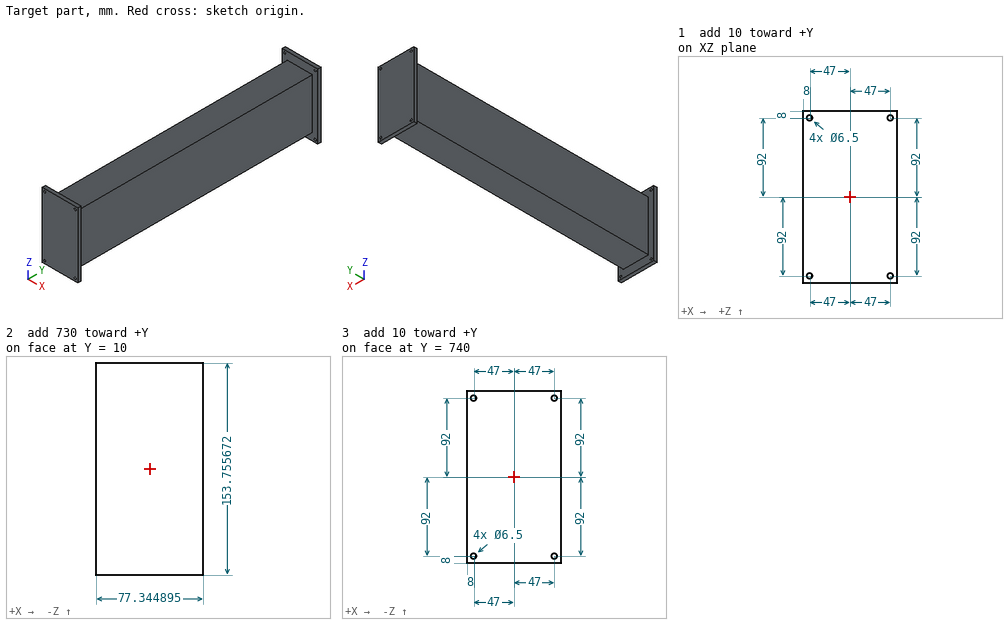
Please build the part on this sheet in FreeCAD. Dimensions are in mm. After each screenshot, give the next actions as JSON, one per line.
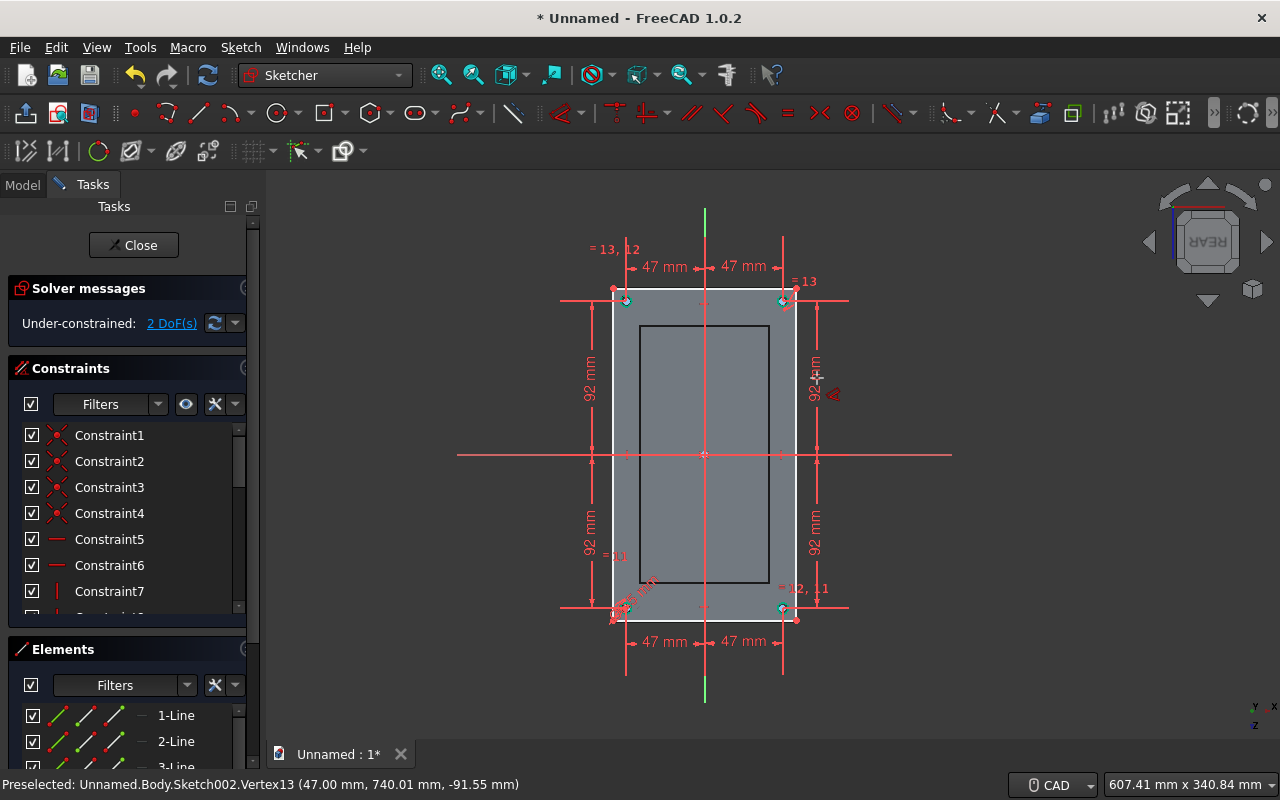
{"action": "scroll", "coordinate": [613, 621], "scroll_direction": "up", "scroll_amount": 6}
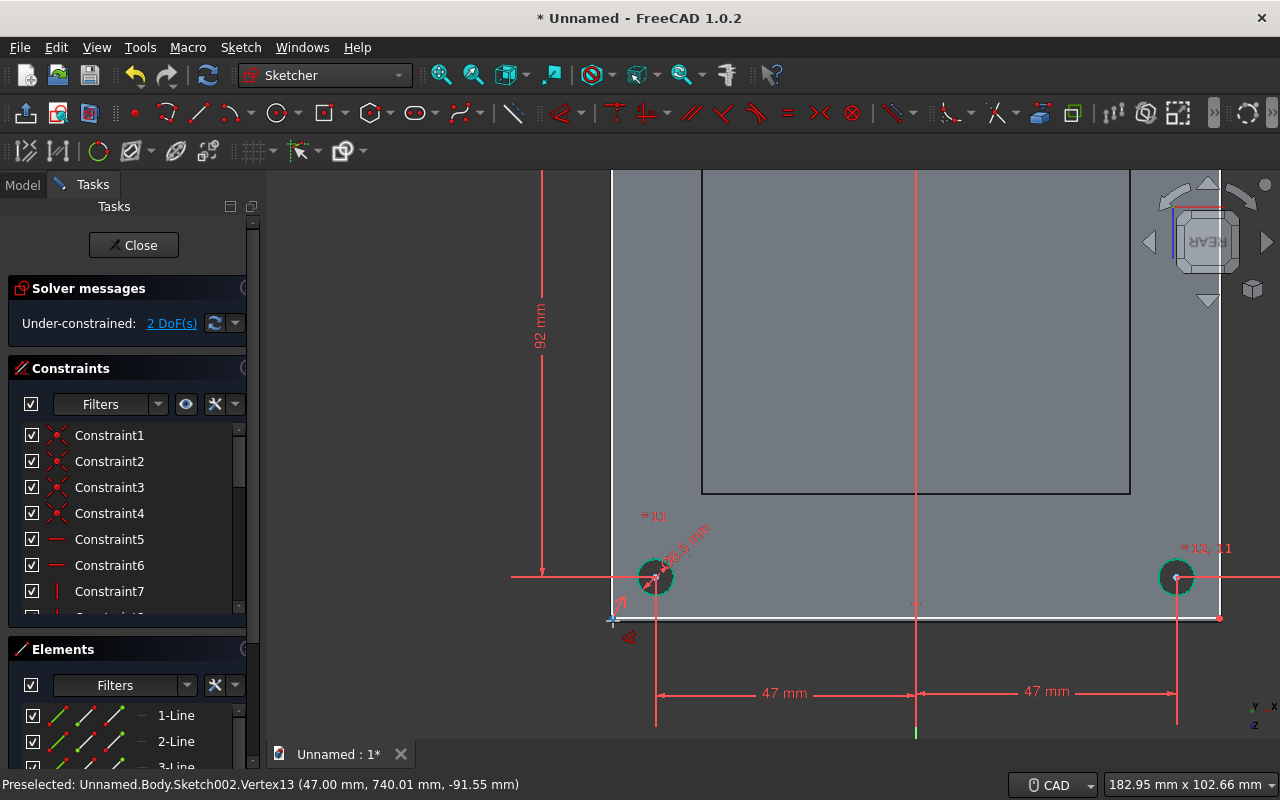
{"action": "left_click", "coordinate": [612, 618]}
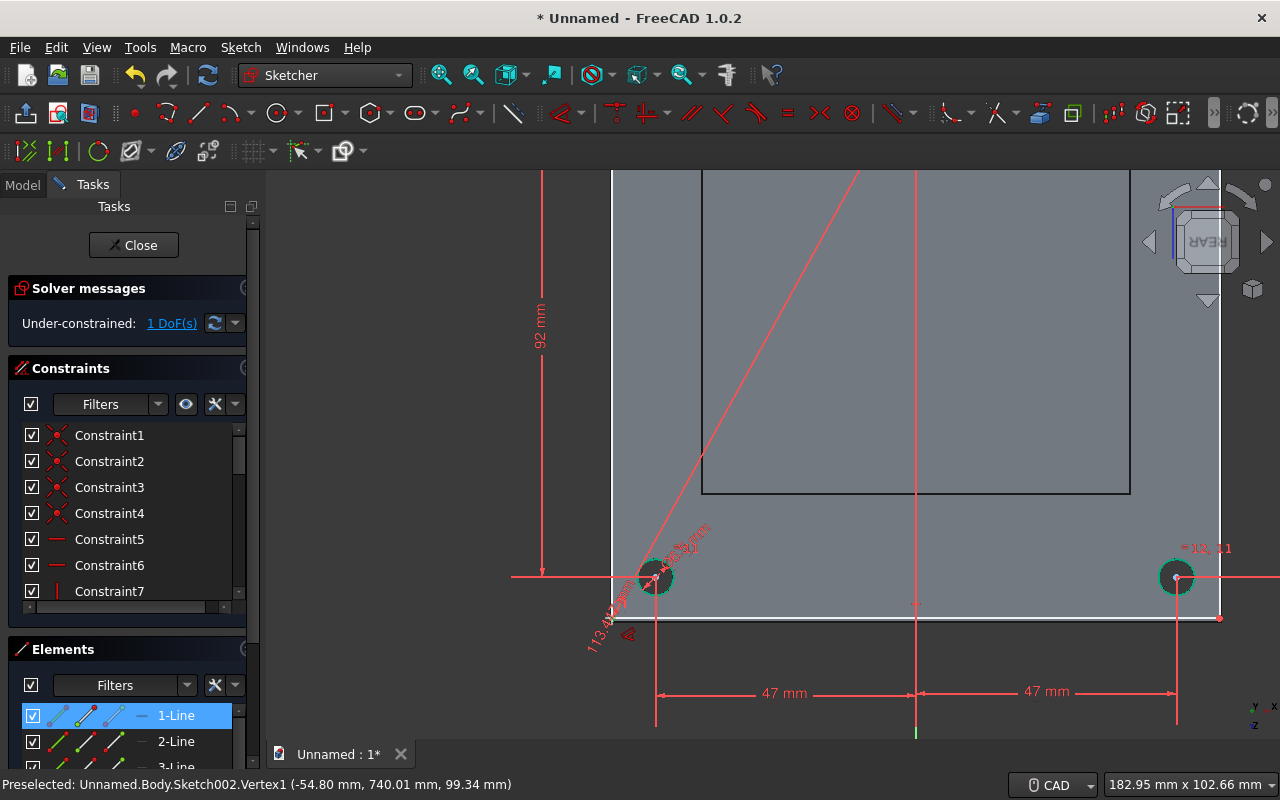
{"action": "left_click", "coordinate": [656, 577]}
{"action": "left_click", "coordinate": [634, 652]}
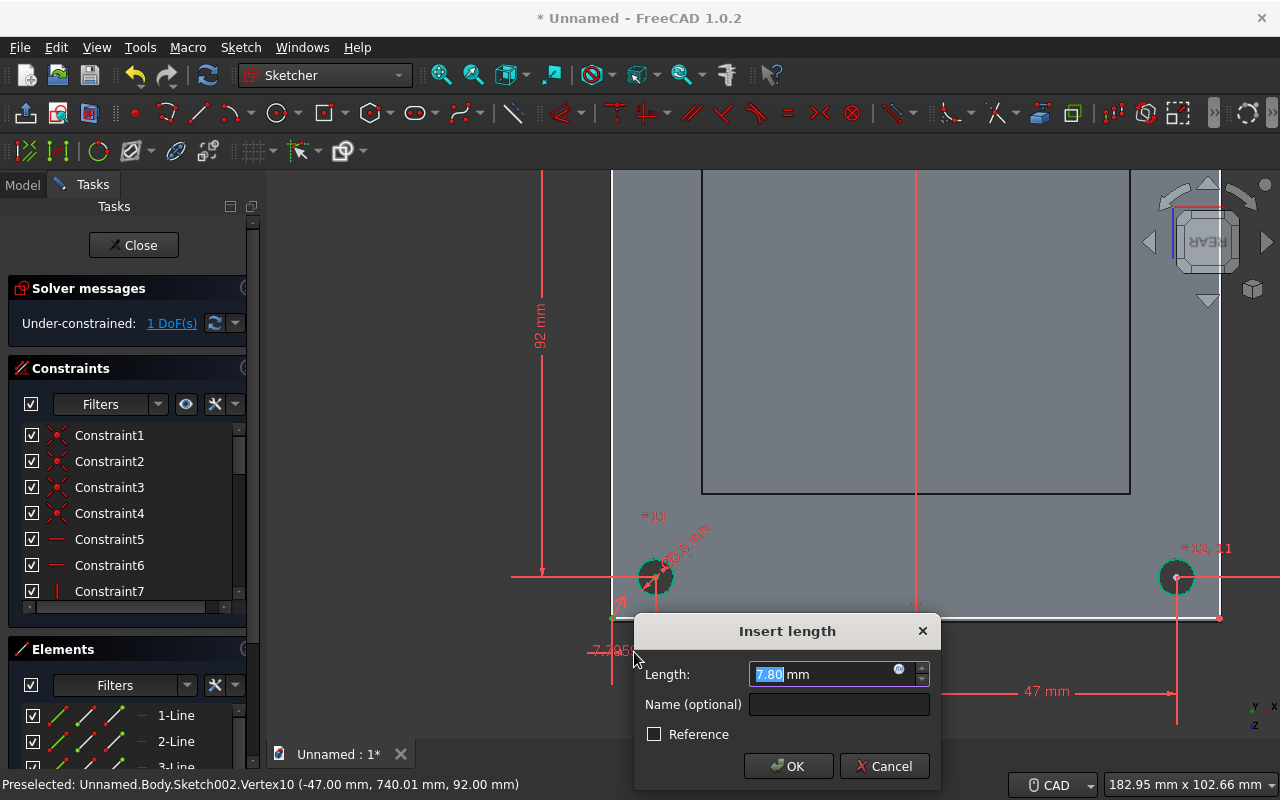
{"action": "type", "text": "8"}
{"action": "key", "text": "Return"}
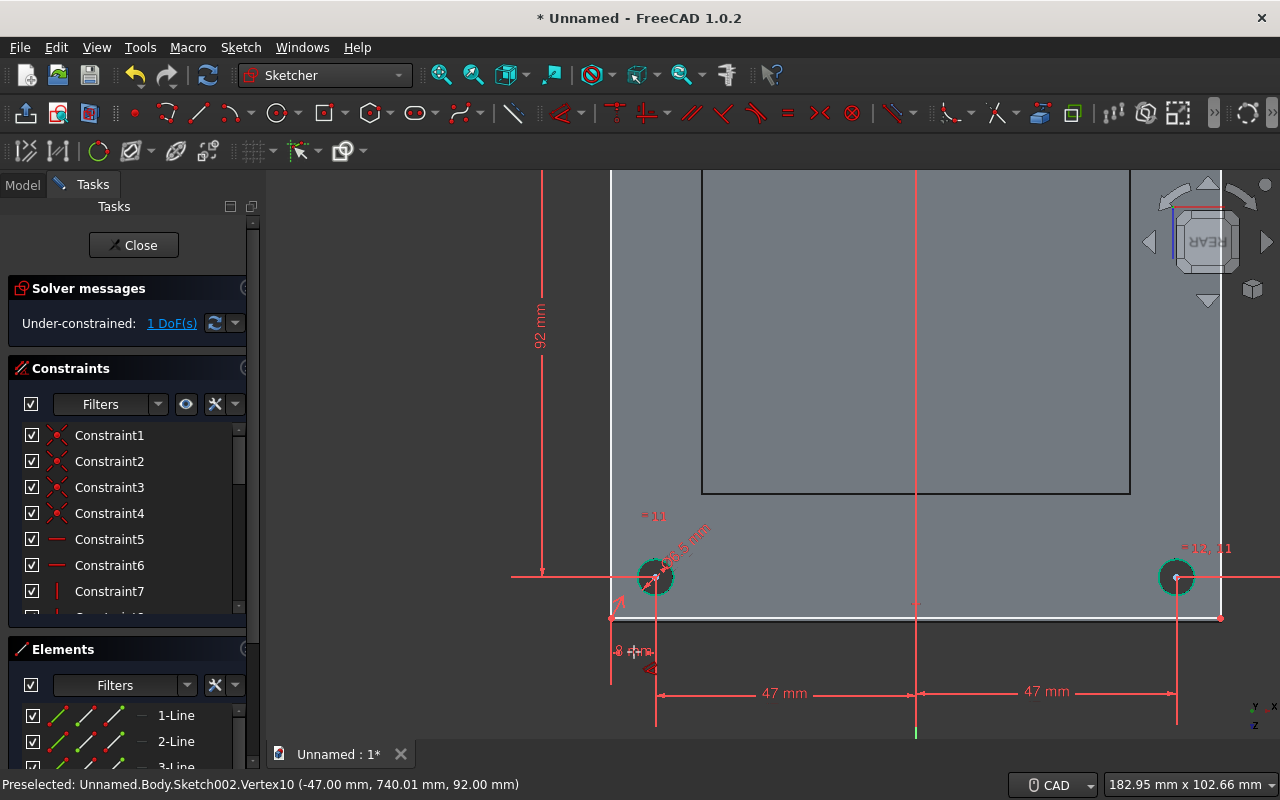
{"action": "left_click", "coordinate": [611, 618]}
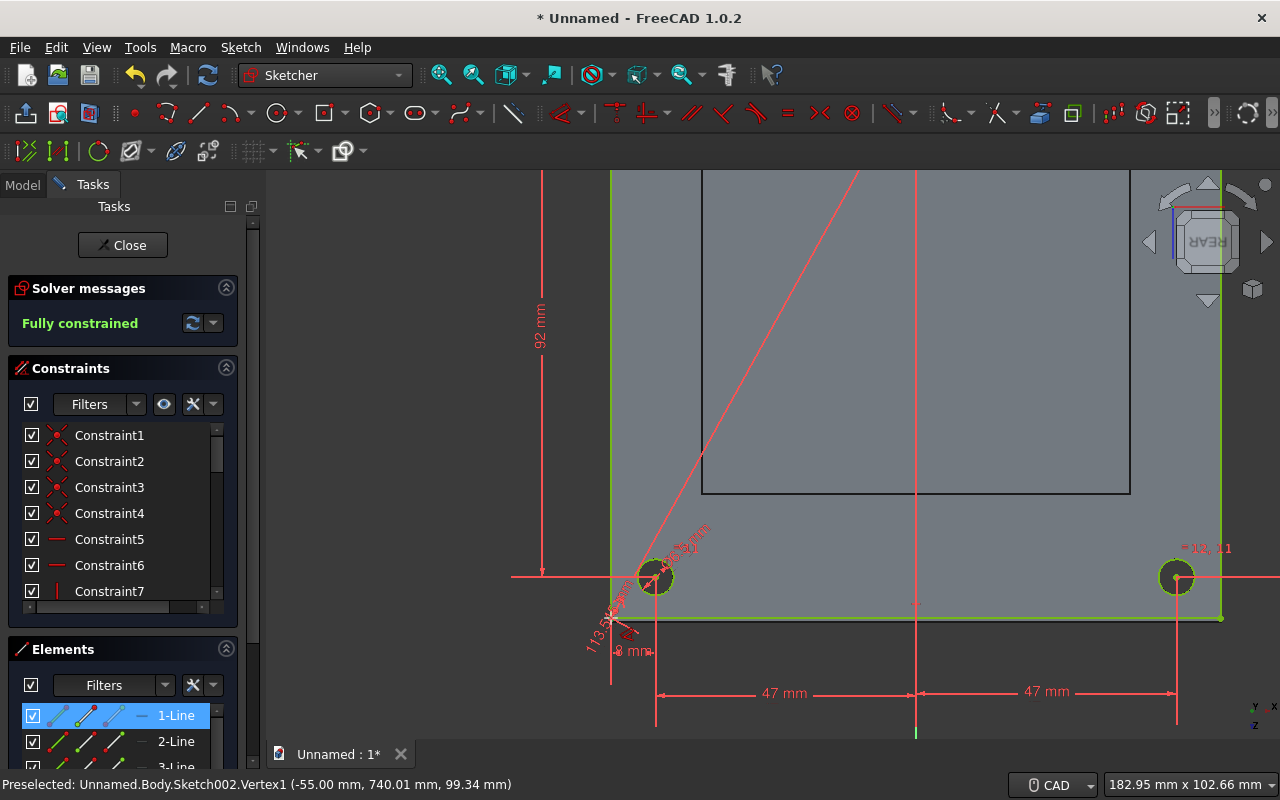
{"action": "left_click", "coordinate": [656, 577]}
{"action": "left_click", "coordinate": [577, 598]}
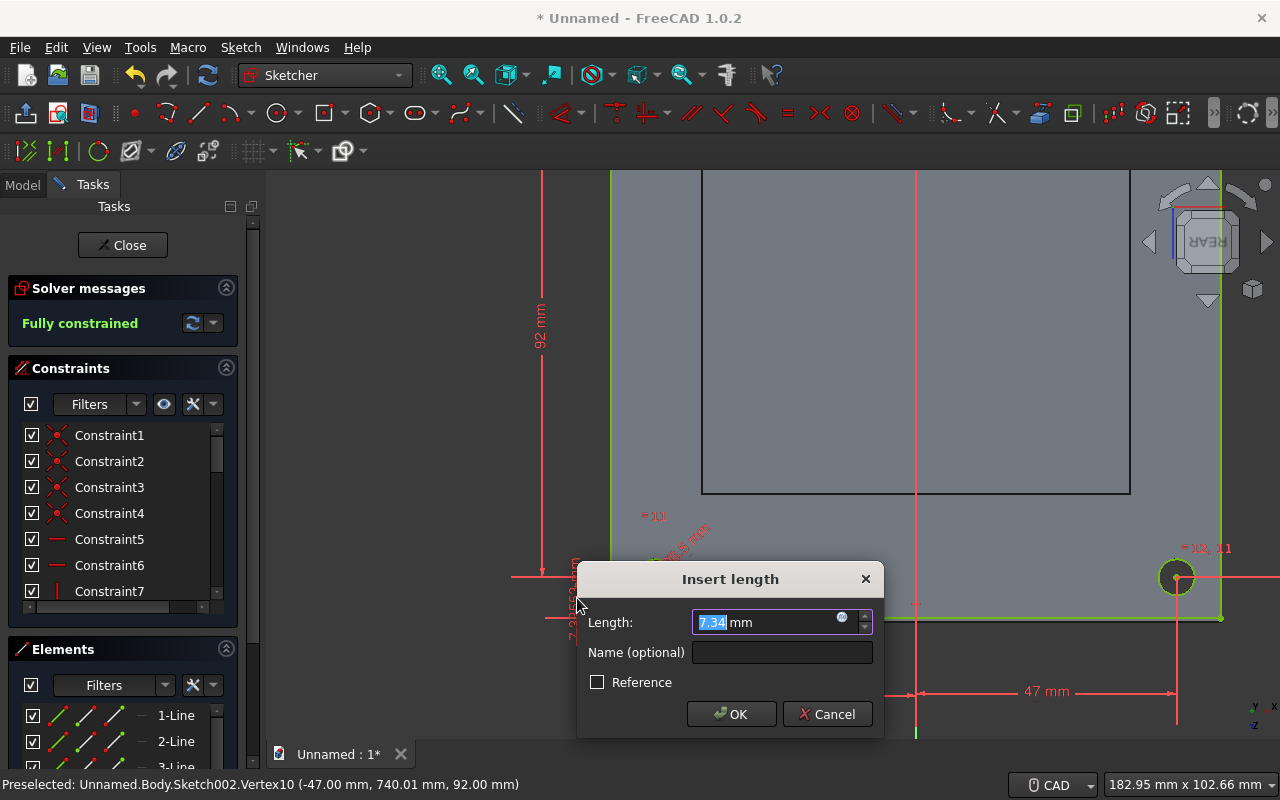
{"action": "type", "text": "8"}
{"action": "key", "text": "Return"}
{"action": "key", "text": "Escape"}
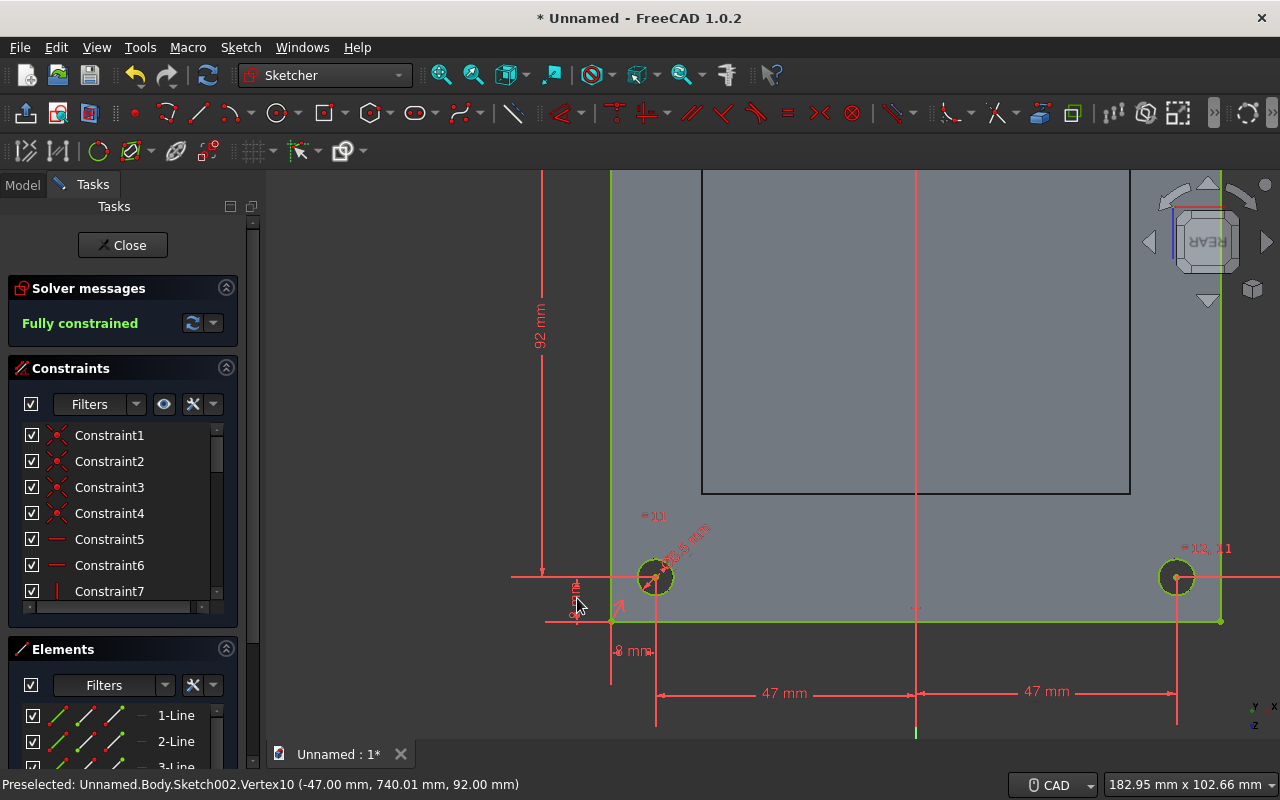
{"action": "left_click", "coordinate": [123, 245]}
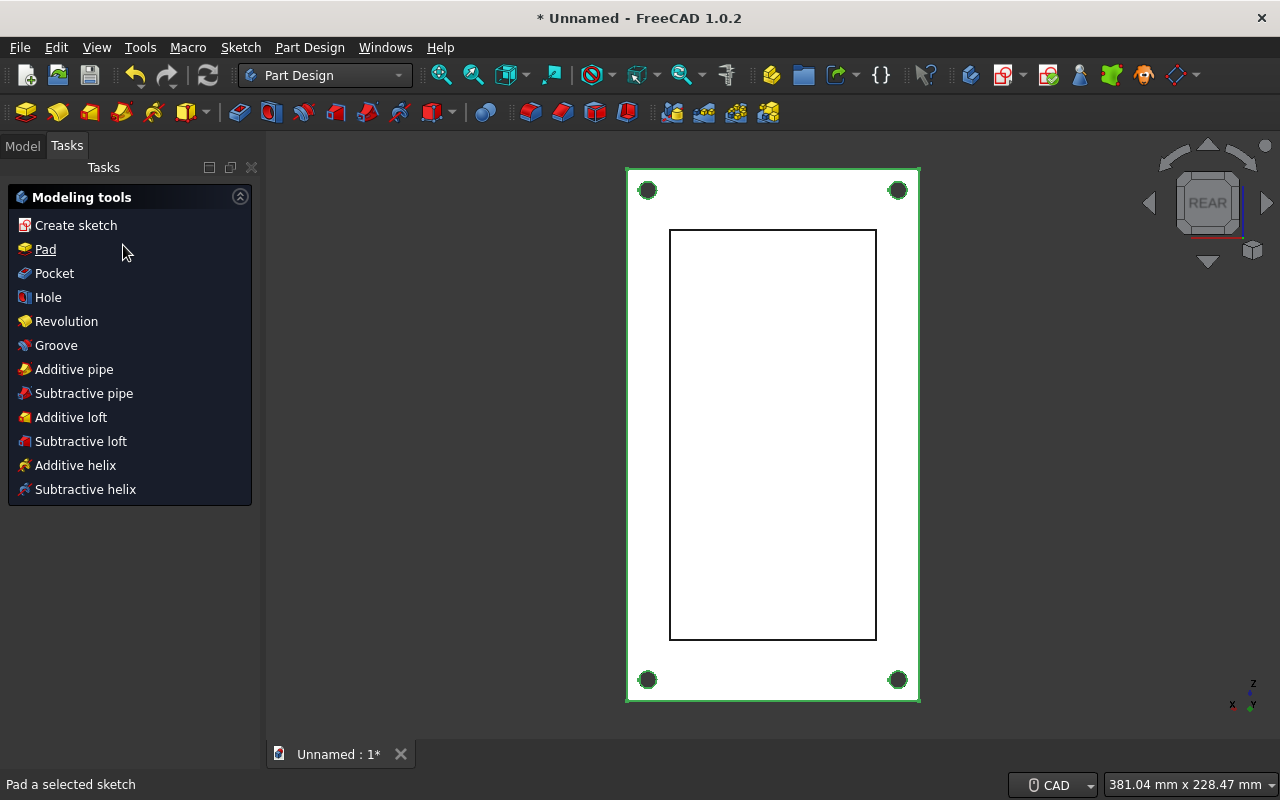
{"action": "left_click", "coordinate": [26, 112]}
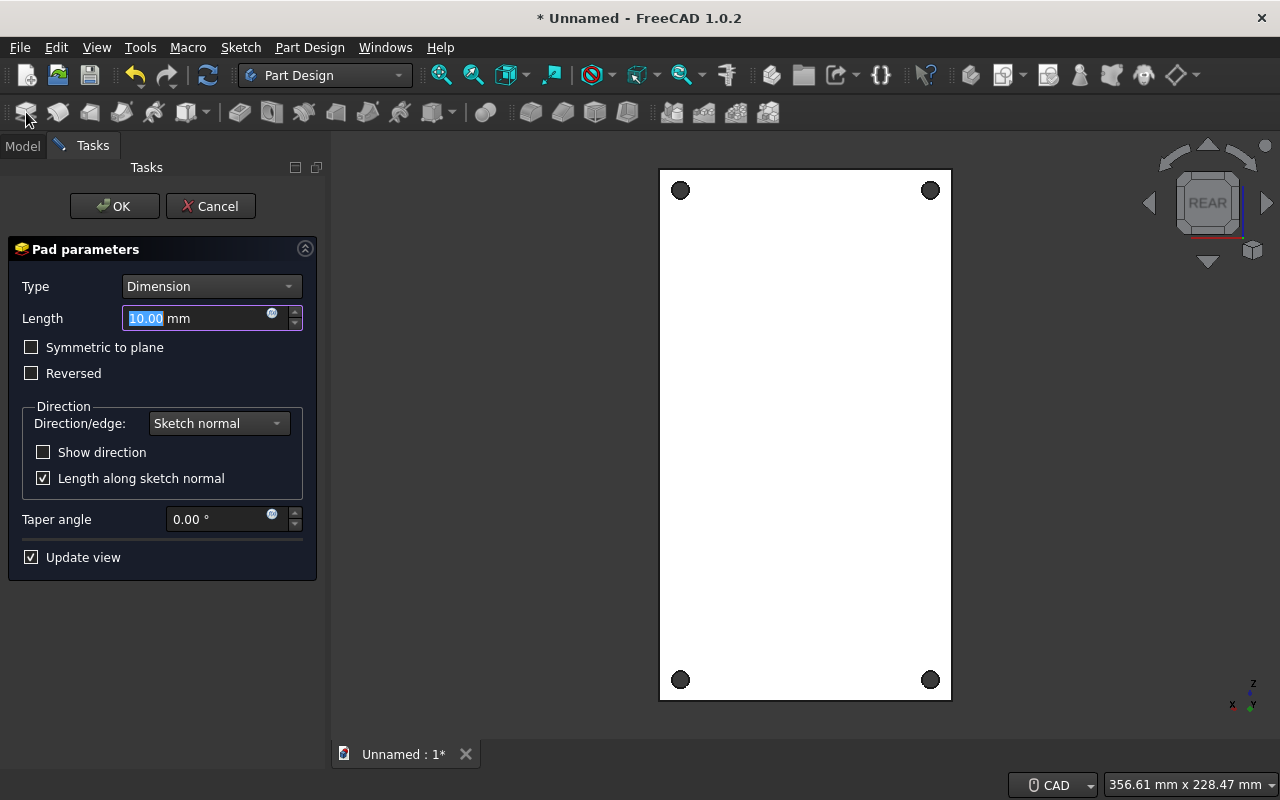
{"action": "type", "text": "10"}
{"action": "key", "text": "Tab"}